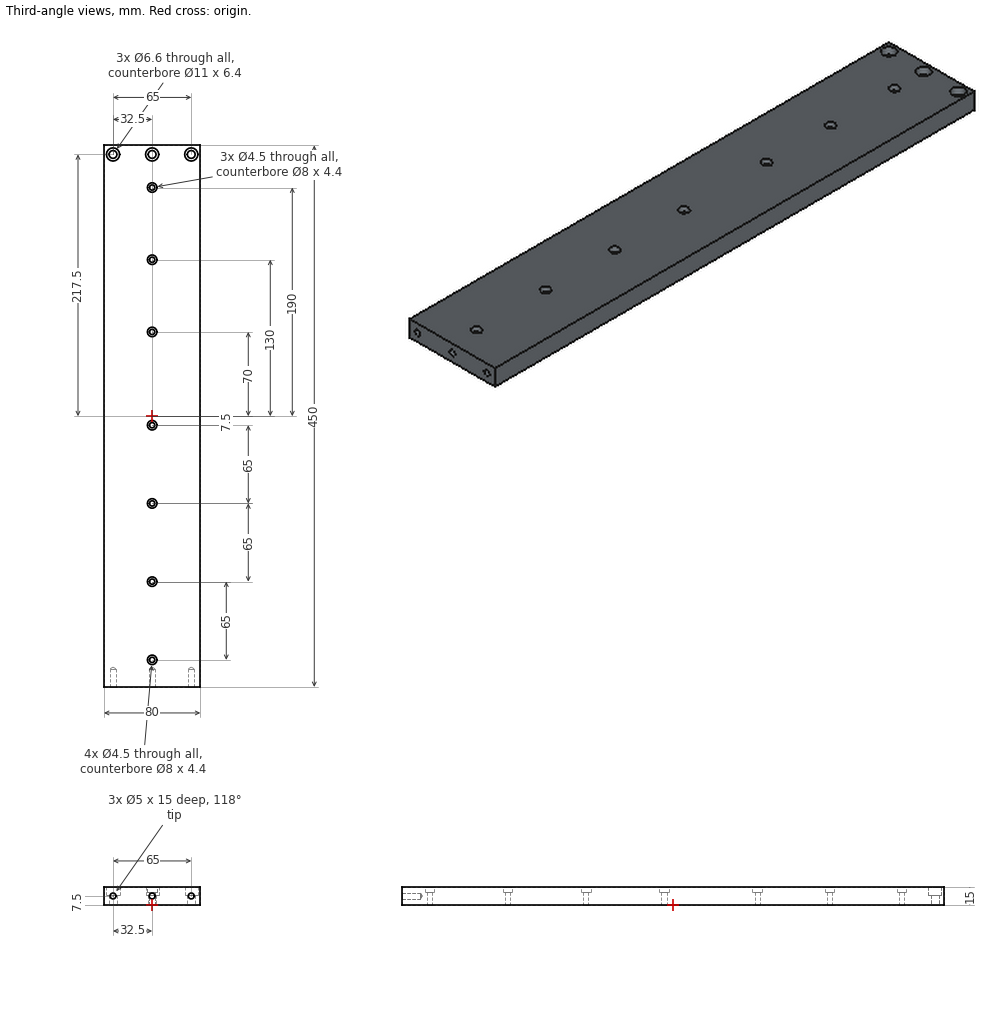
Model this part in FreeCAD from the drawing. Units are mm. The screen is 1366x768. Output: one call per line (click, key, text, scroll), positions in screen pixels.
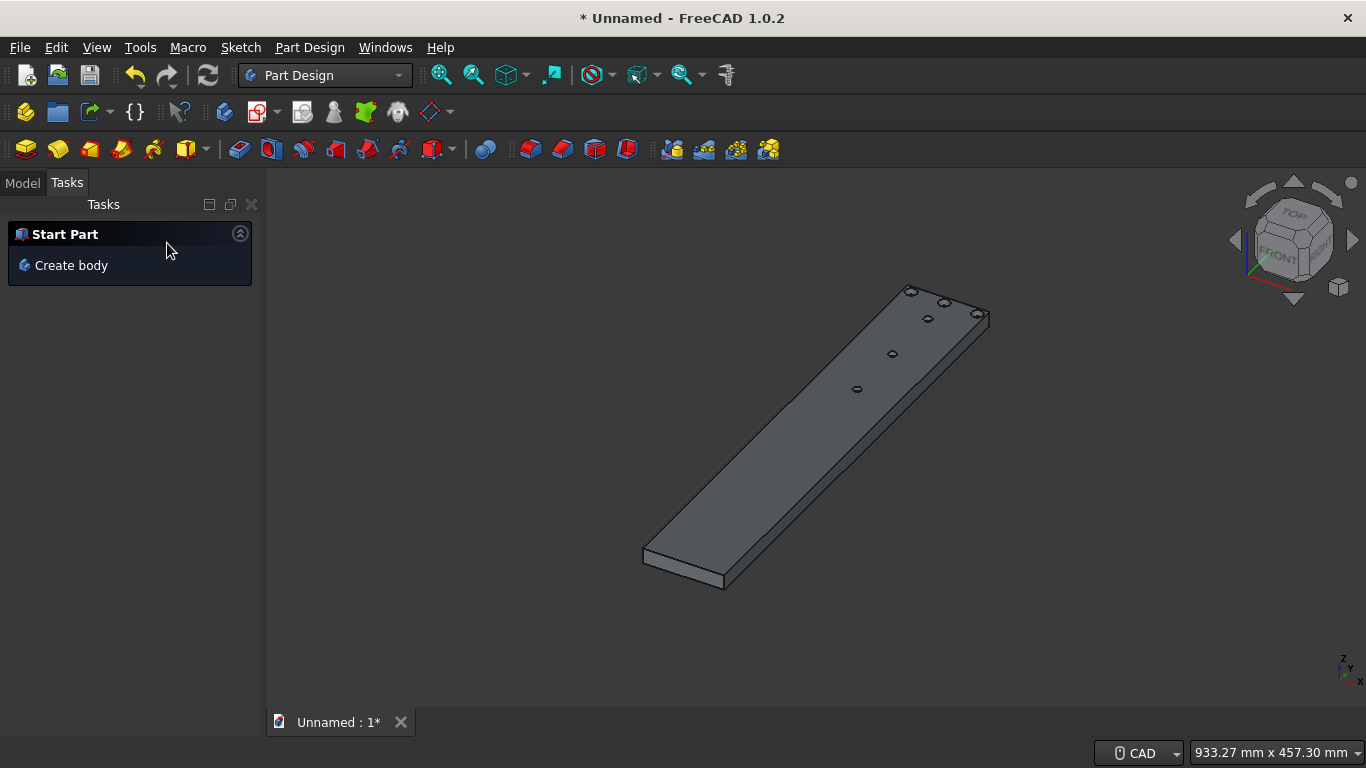
click(816, 429)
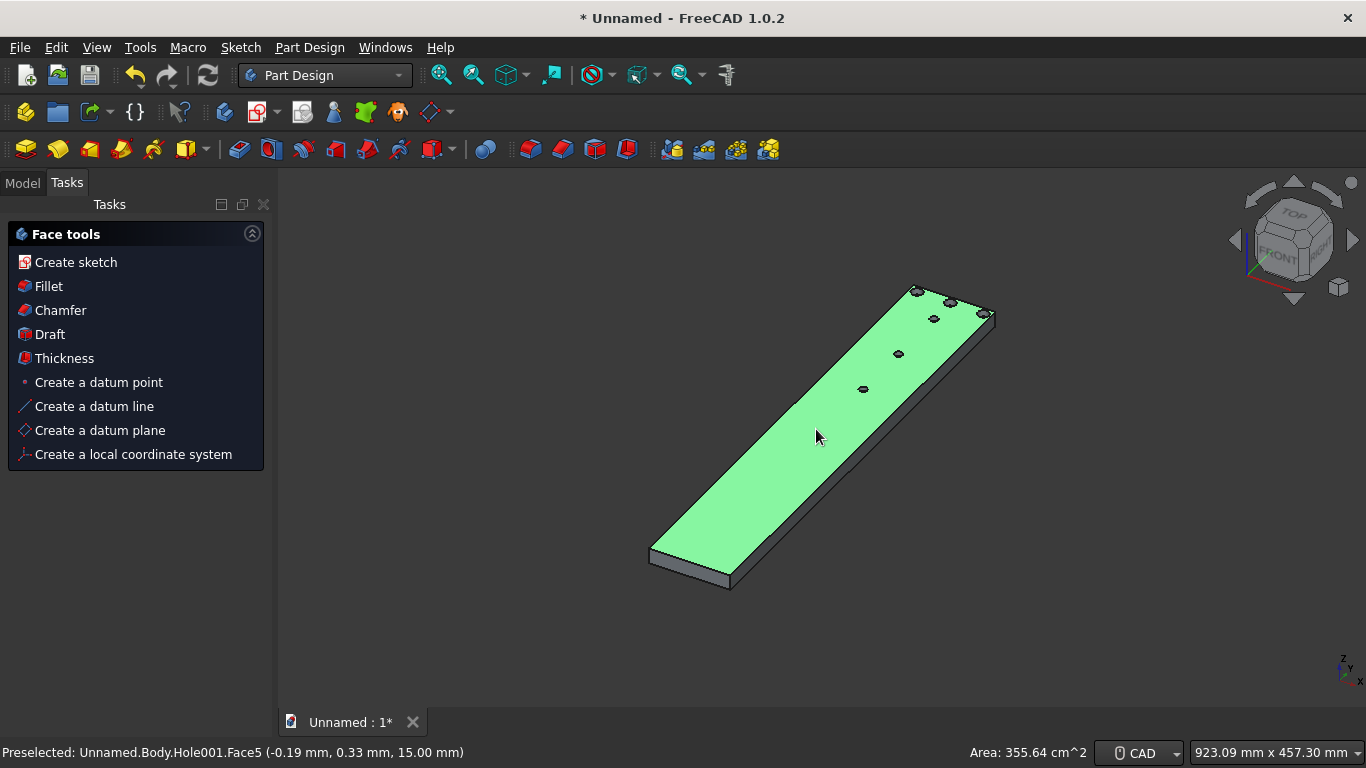
click(258, 112)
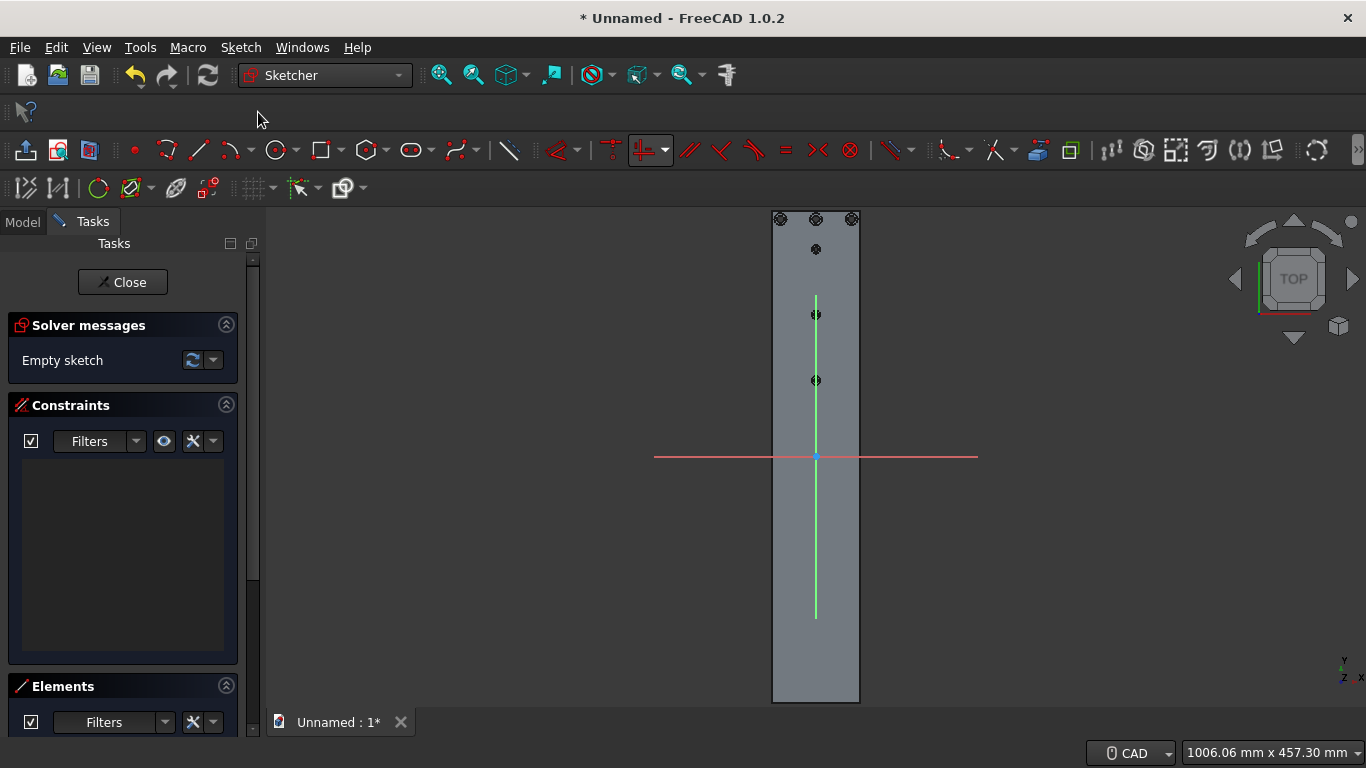
scroll(438, 235, down, 1)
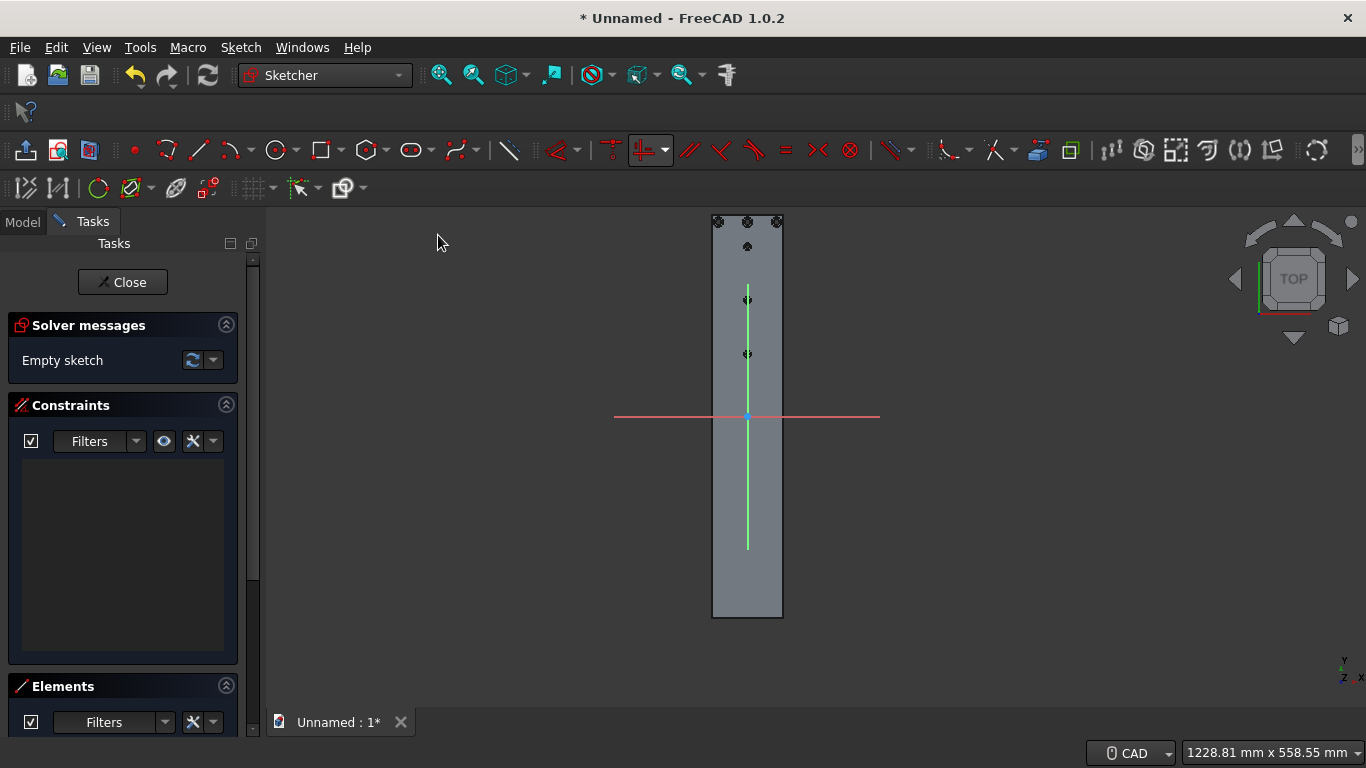
scroll(748, 571, up, 3)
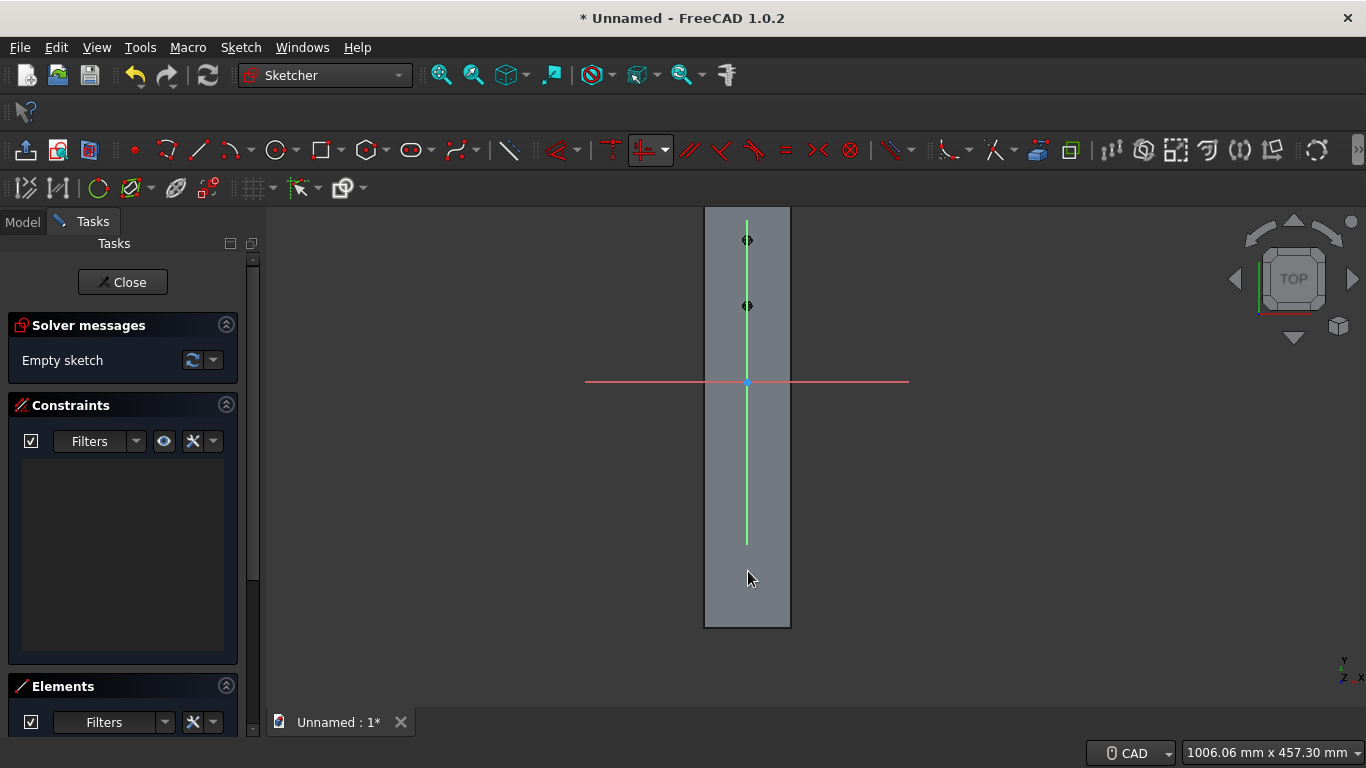
click(276, 150)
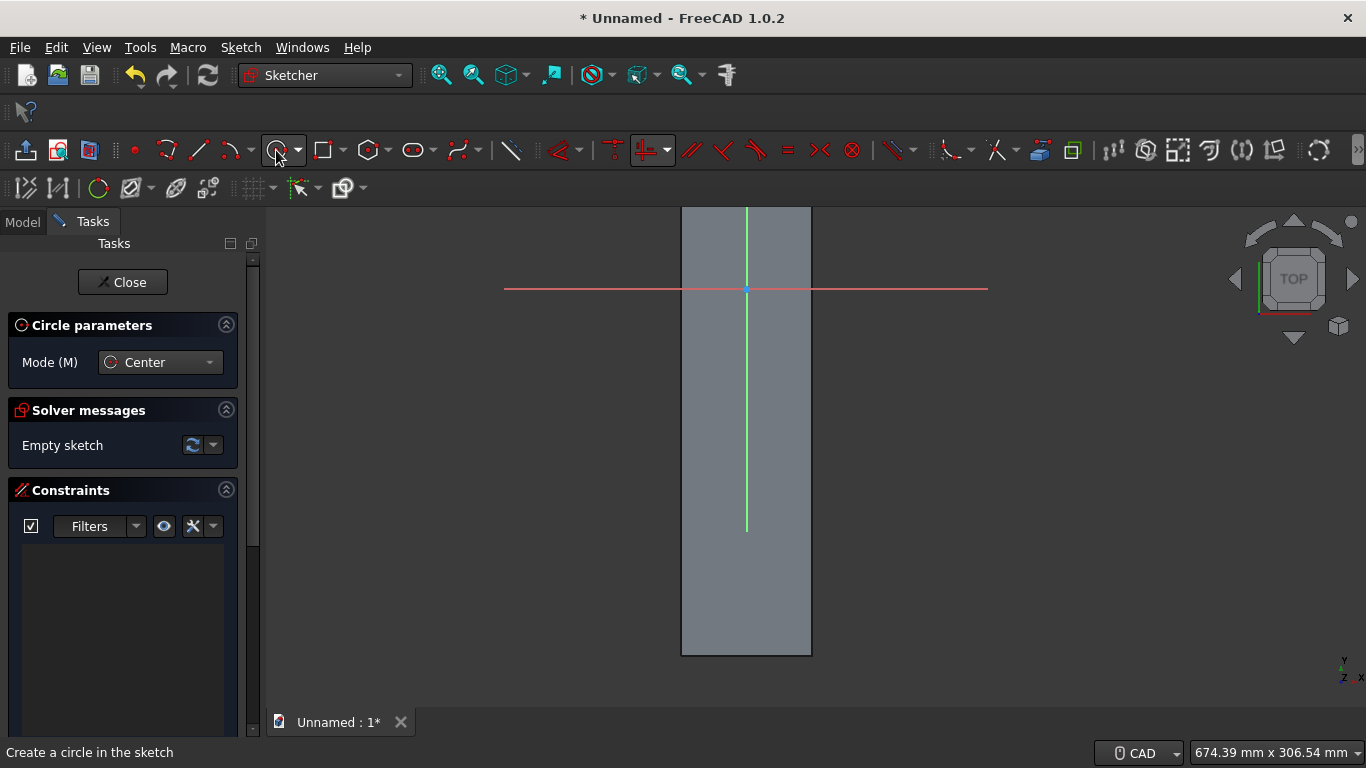
scroll(747, 620, up, 10)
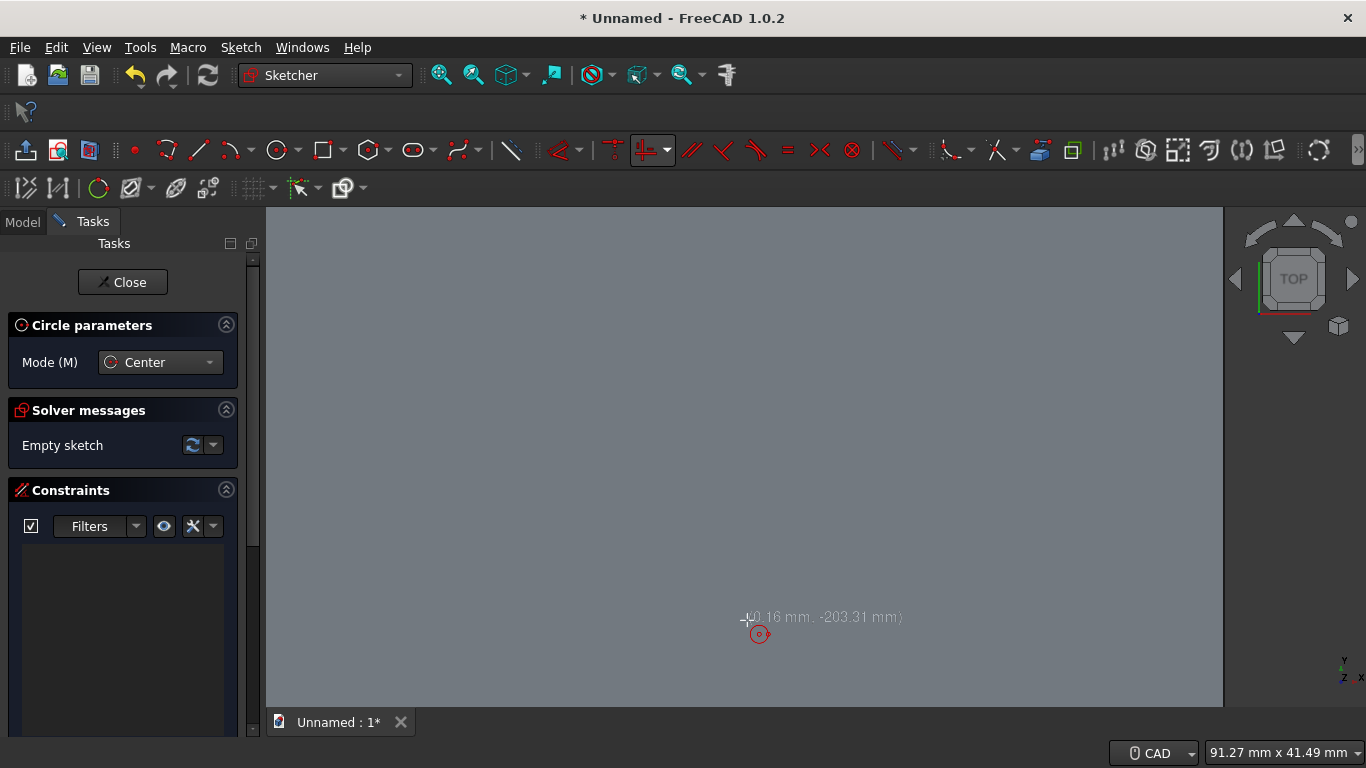
scroll(748, 622, down, 10)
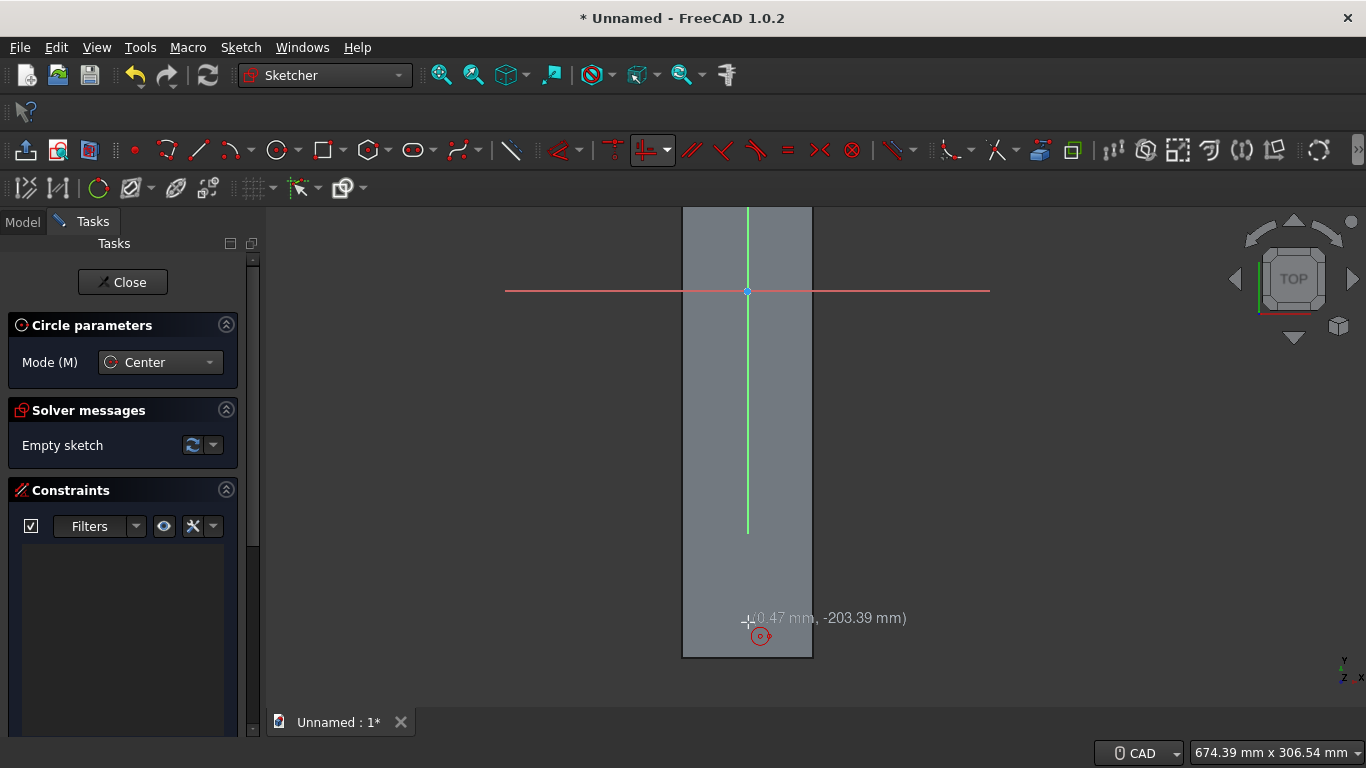
click(748, 621)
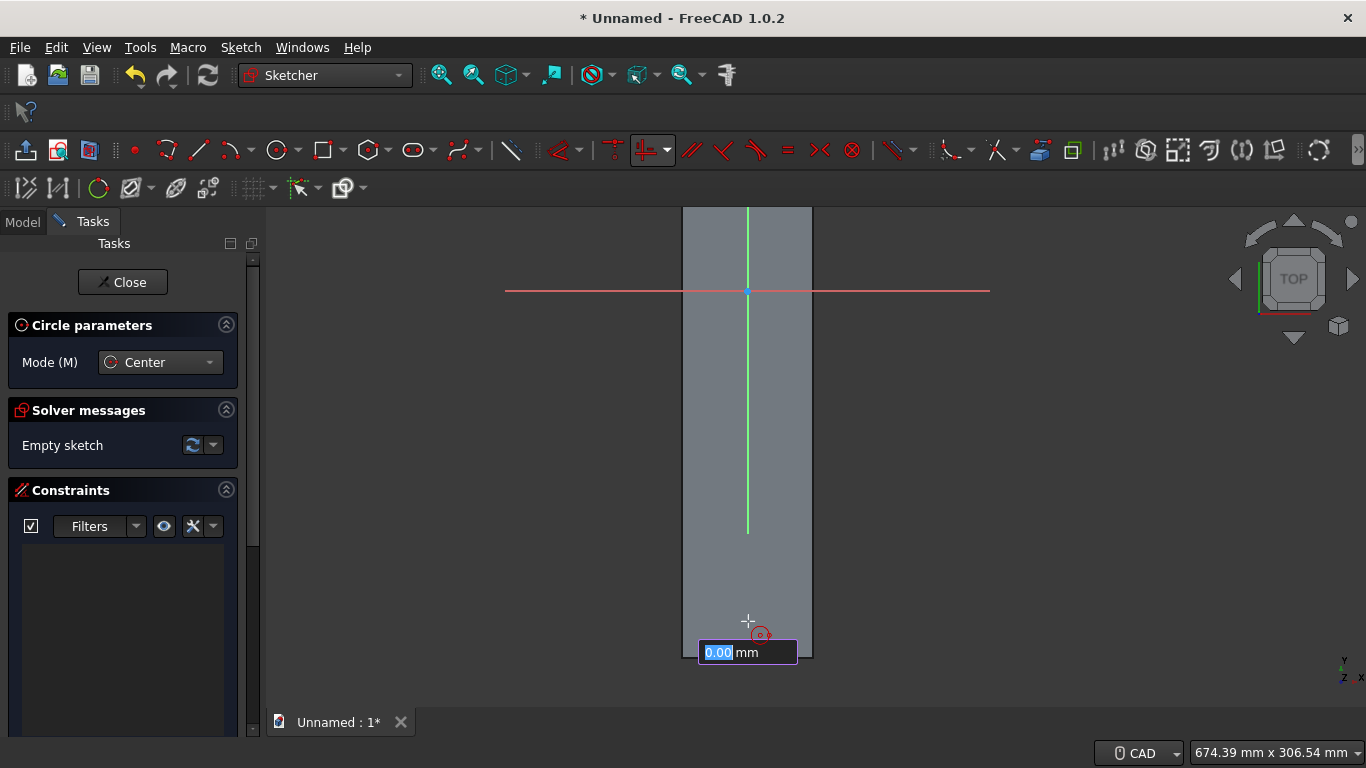
scroll(751, 620, up, 8)
move(750, 617)